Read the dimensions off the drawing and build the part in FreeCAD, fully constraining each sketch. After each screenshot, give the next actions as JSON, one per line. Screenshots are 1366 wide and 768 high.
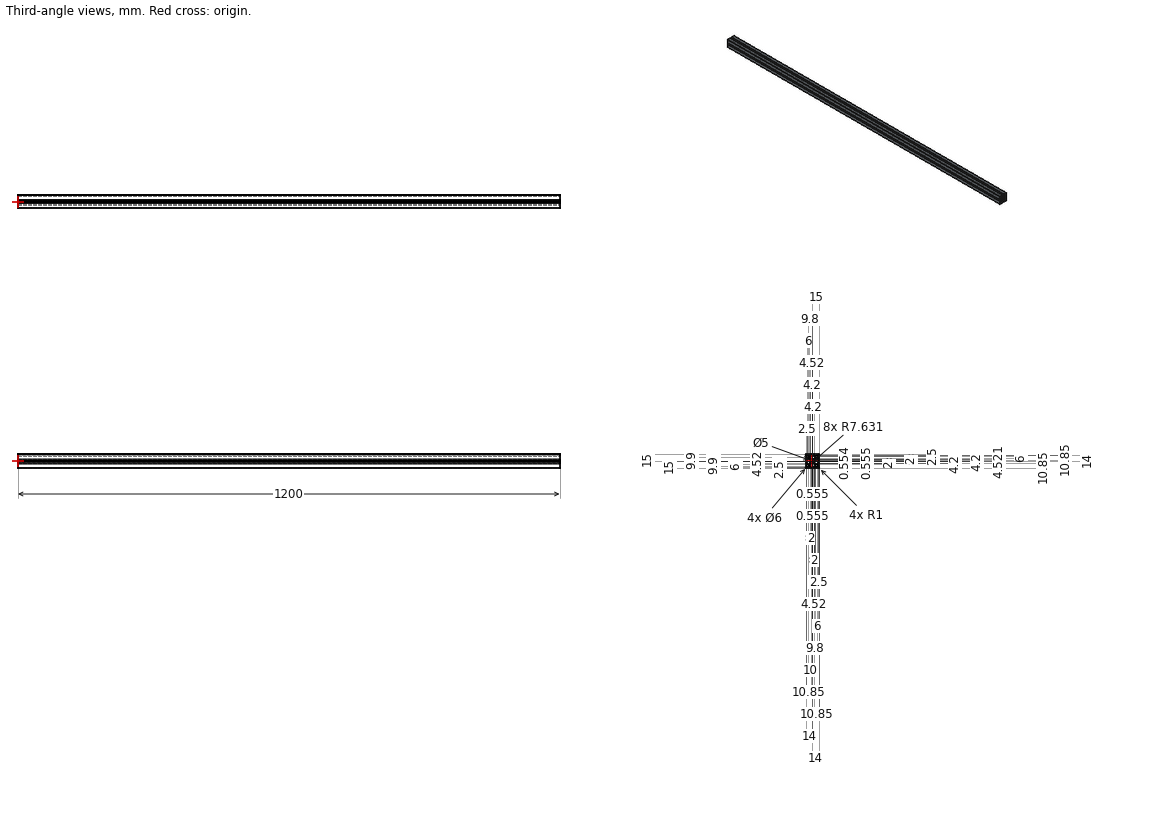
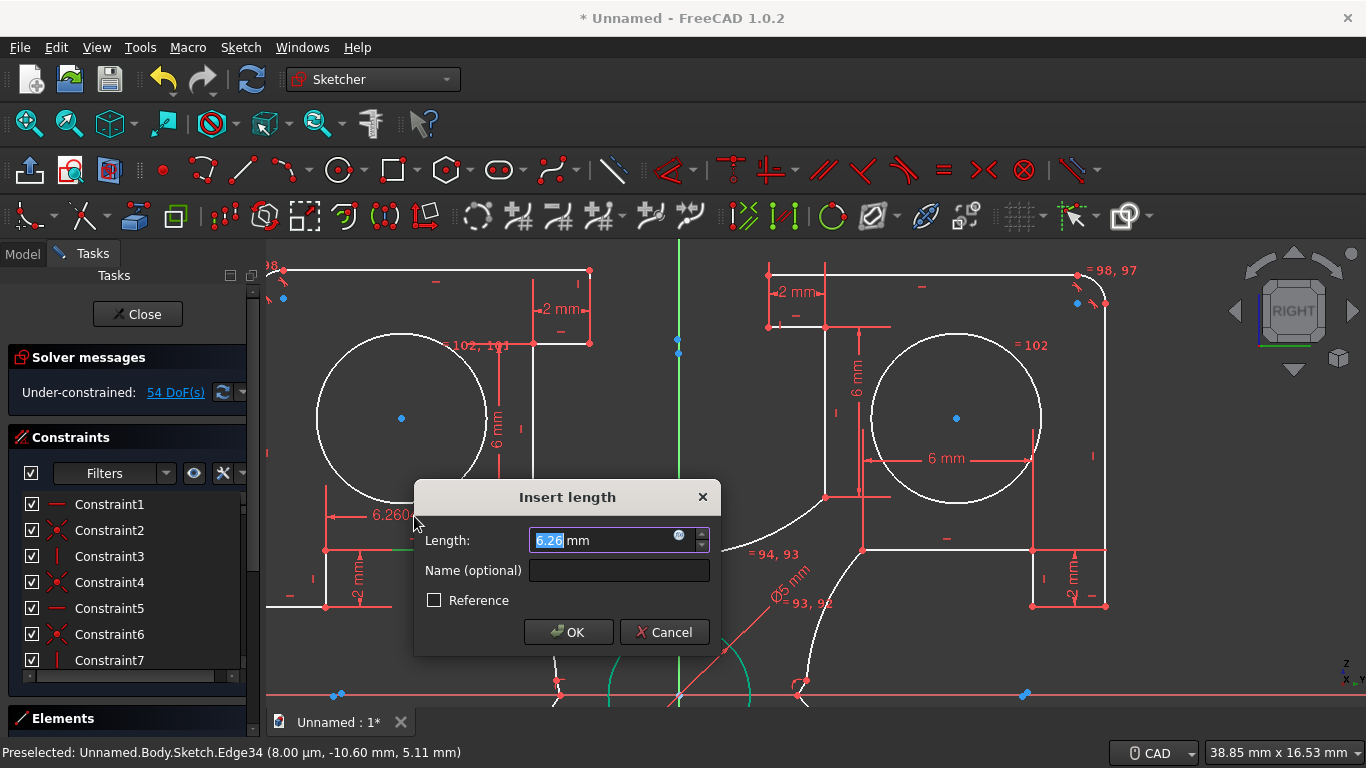
{"action": "type", "text": "6"}
{"action": "key", "text": "Return"}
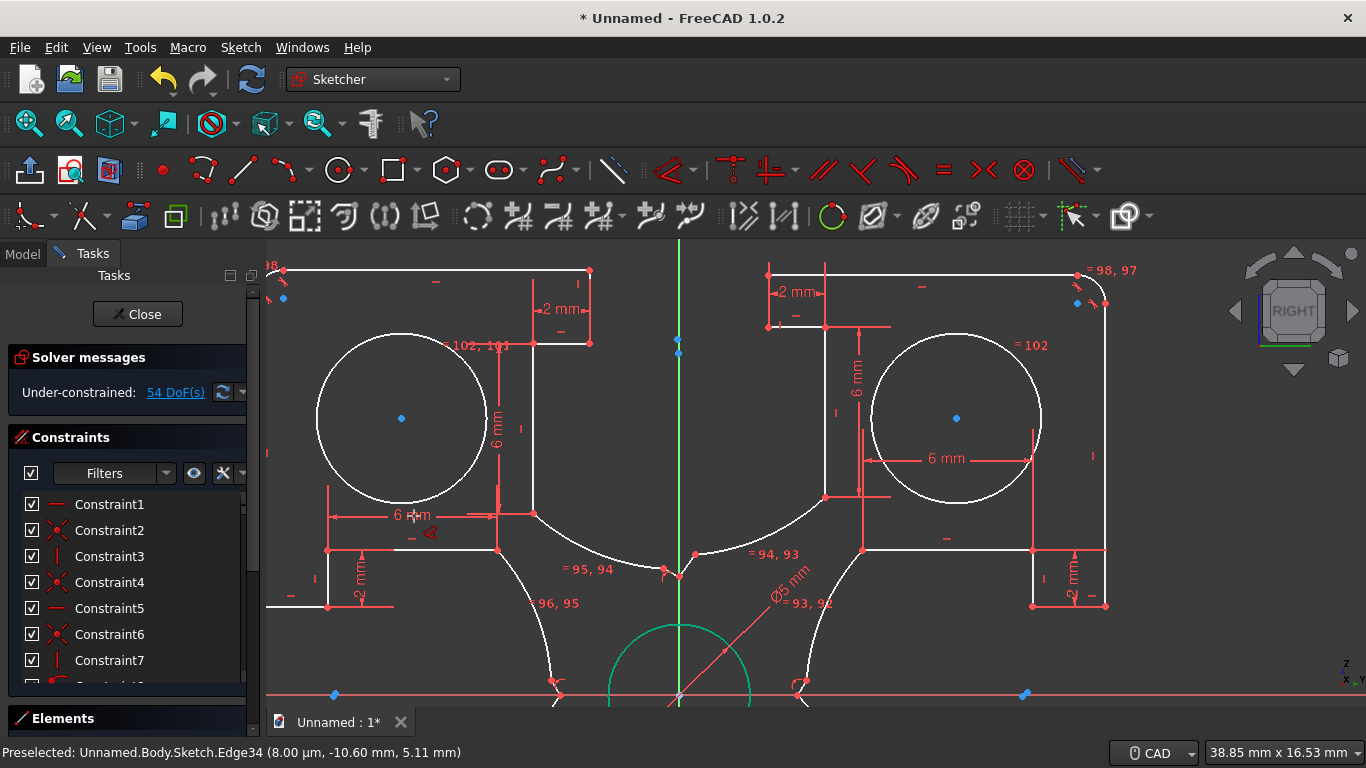
{"action": "scroll", "coordinate": [787, 344], "scroll_direction": "down", "scroll_amount": 5}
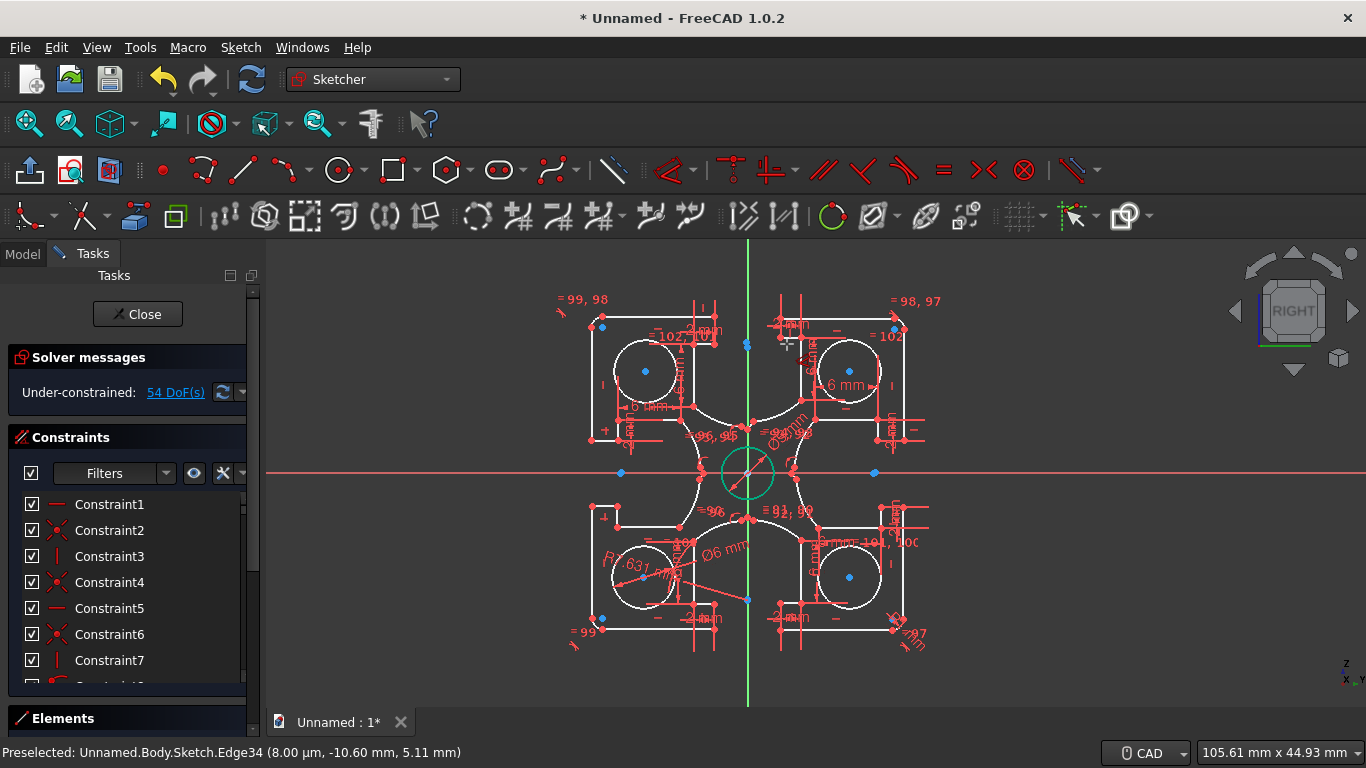
{"action": "left_click", "coordinate": [661, 527]}
{"action": "left_click", "coordinate": [648, 493]}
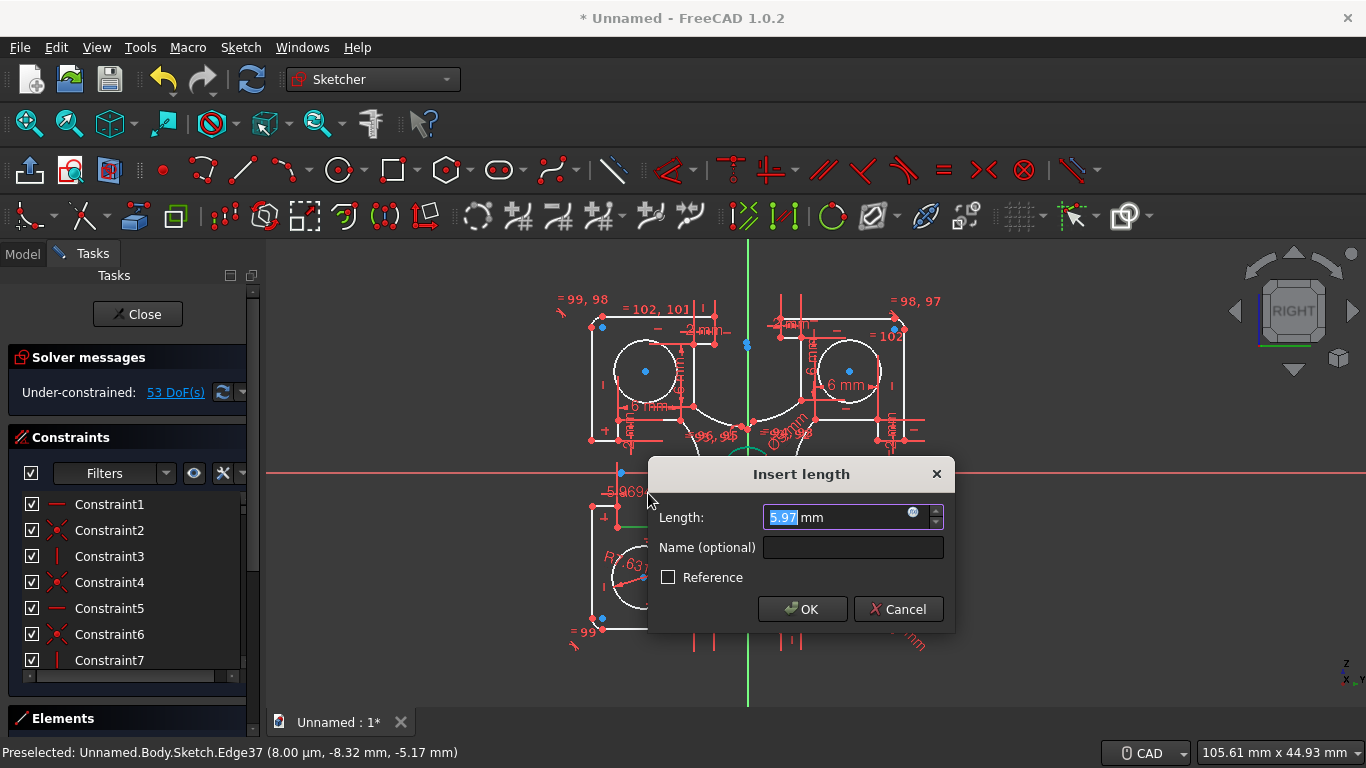
{"action": "type", "text": "6"}
{"action": "key", "text": "Return"}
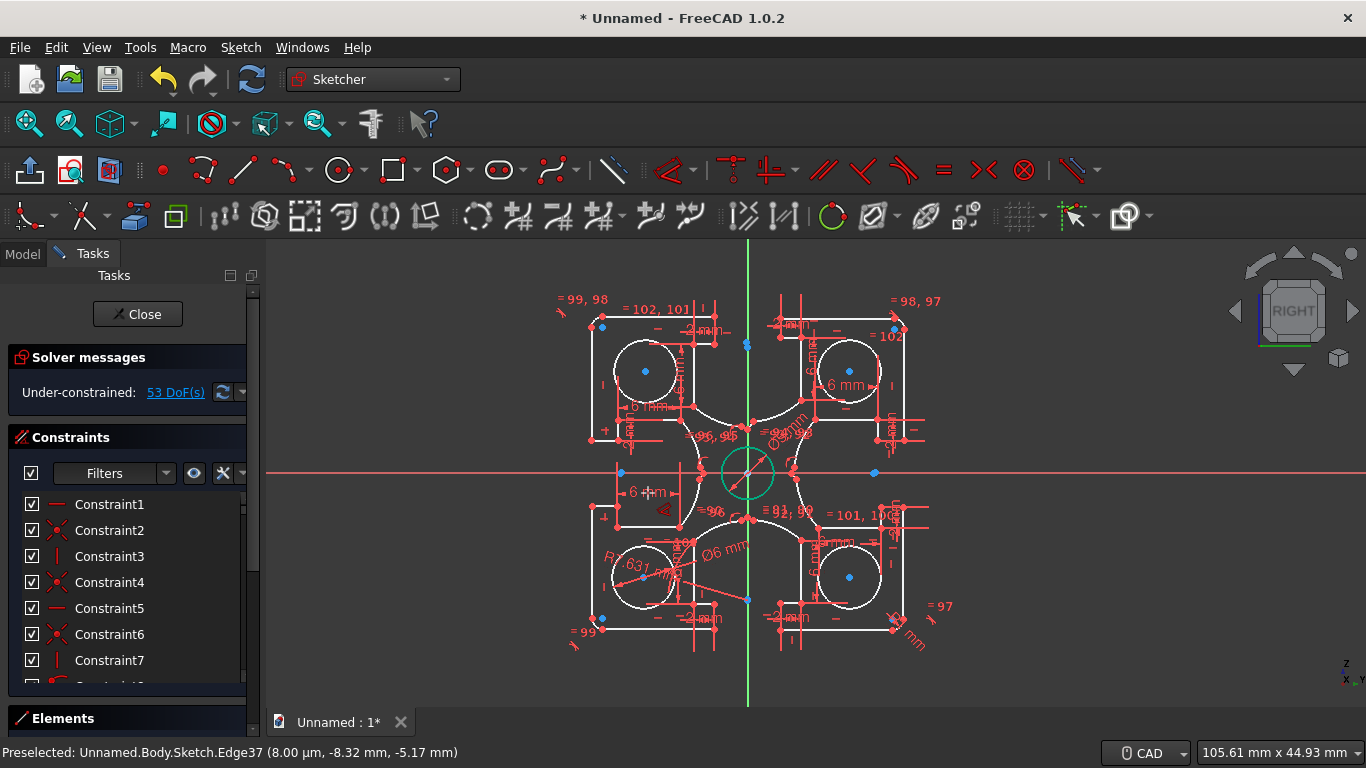
{"action": "scroll", "coordinate": [617, 517], "scroll_direction": "up", "scroll_amount": 4}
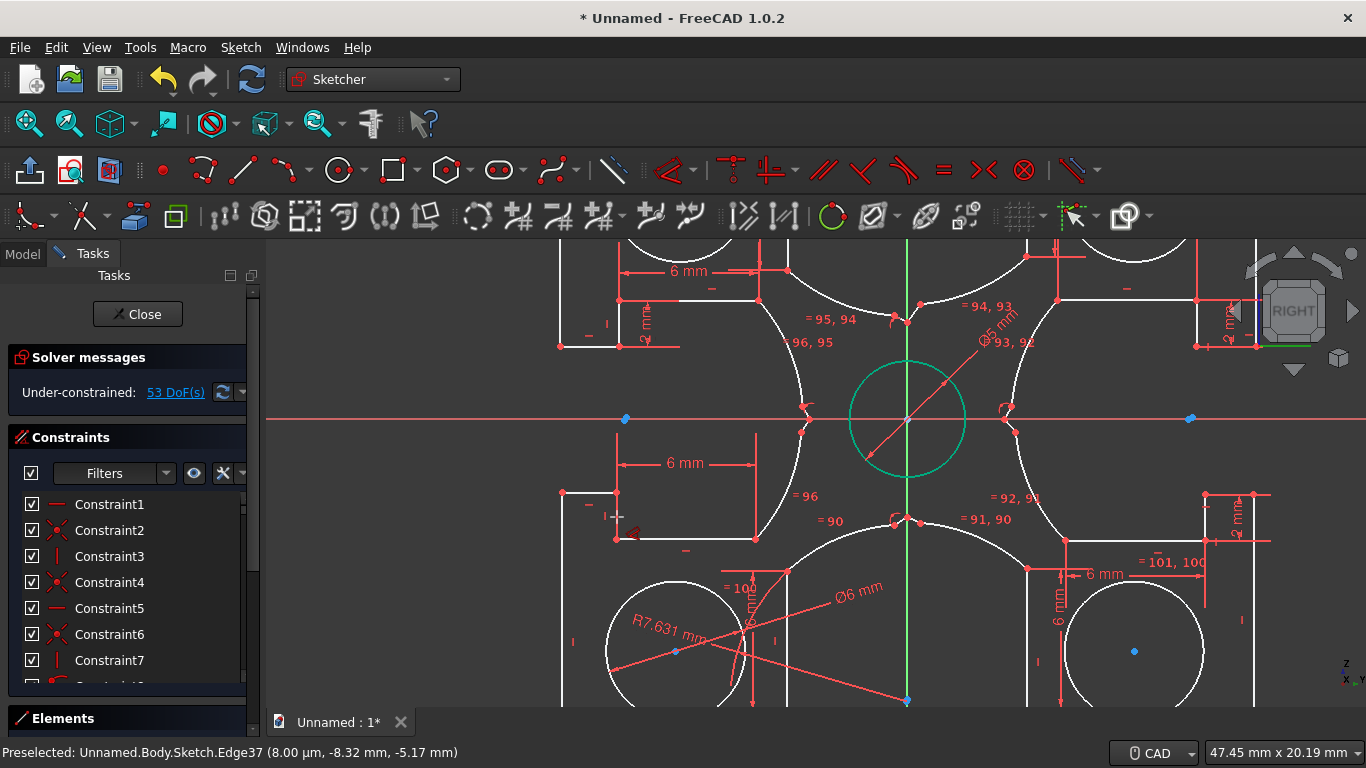
{"action": "left_click", "coordinate": [617, 516]}
{"action": "left_click", "coordinate": [583, 516]}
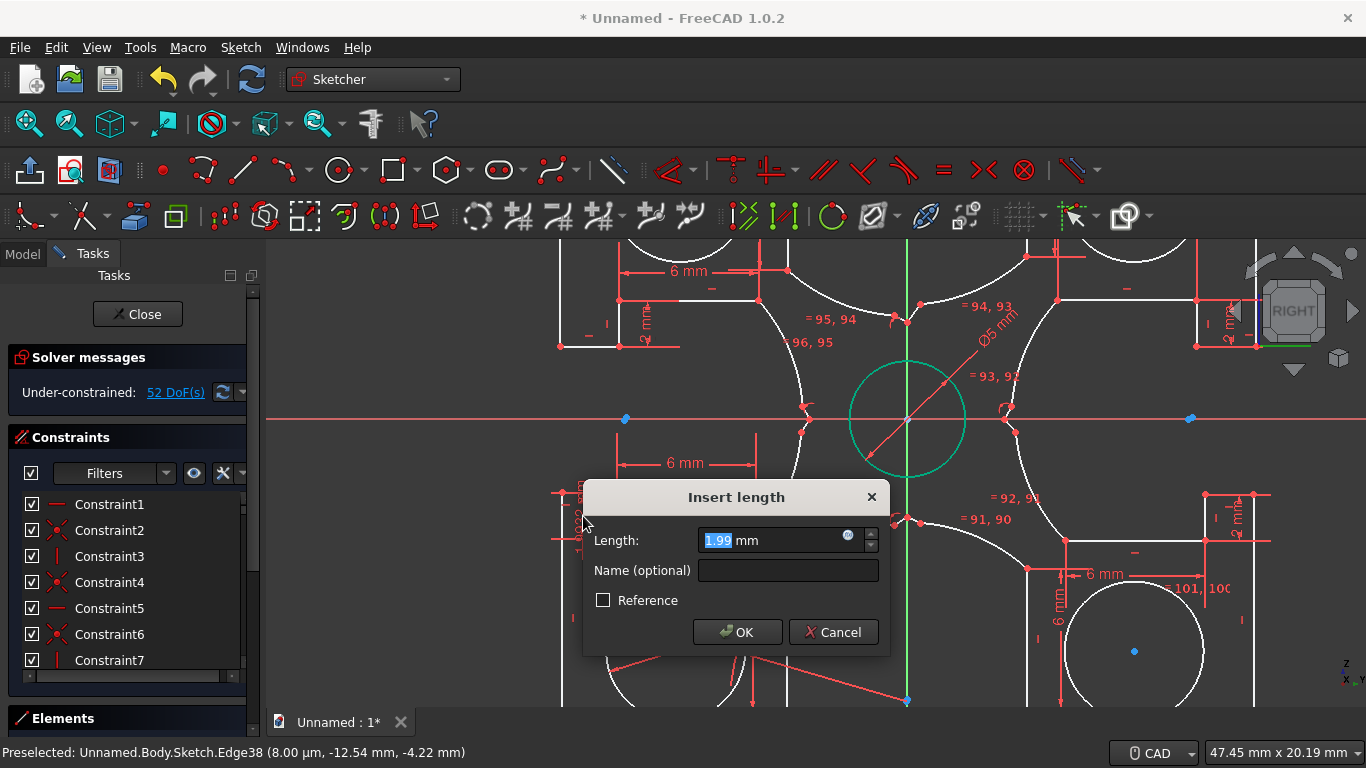
{"action": "type", "text": "2"}
{"action": "key", "text": "Return"}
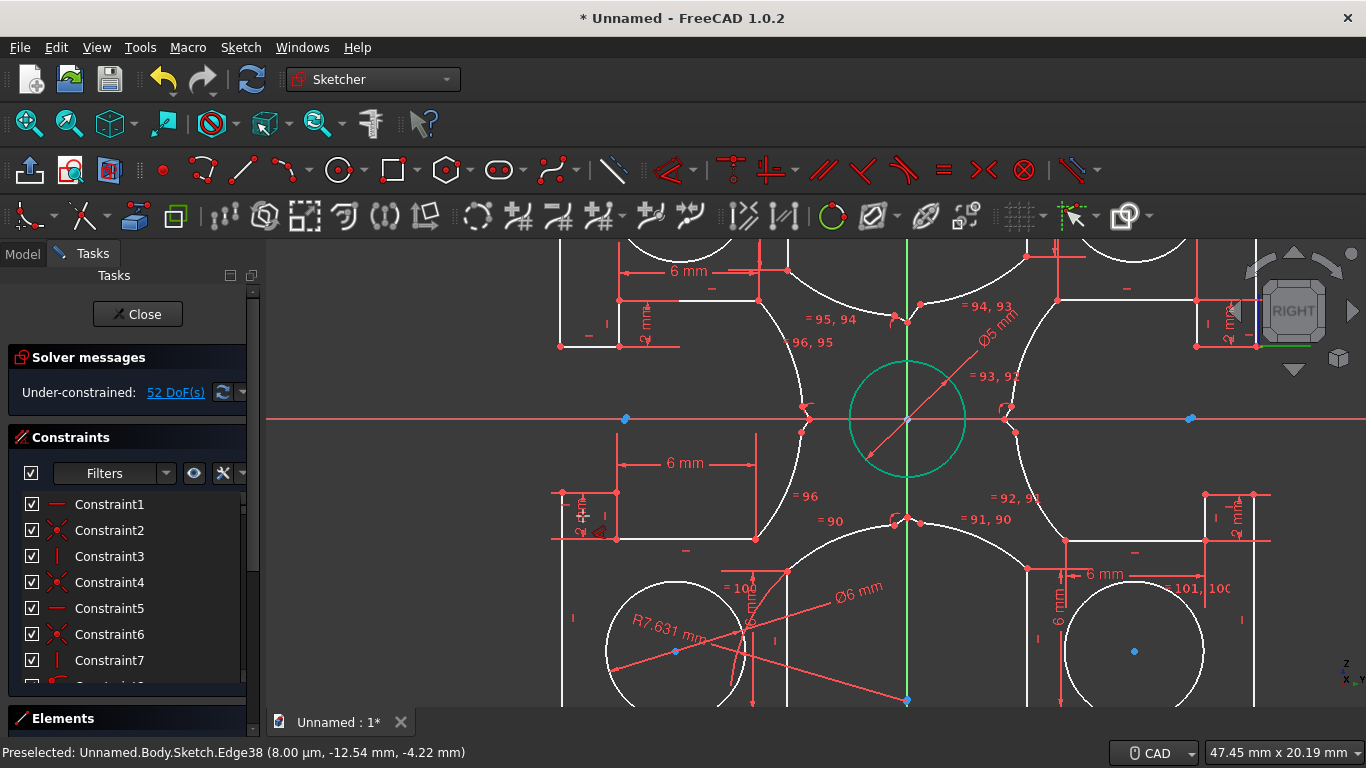
{"action": "left_click", "coordinate": [676, 651]}
{"action": "left_click", "coordinate": [738, 385]}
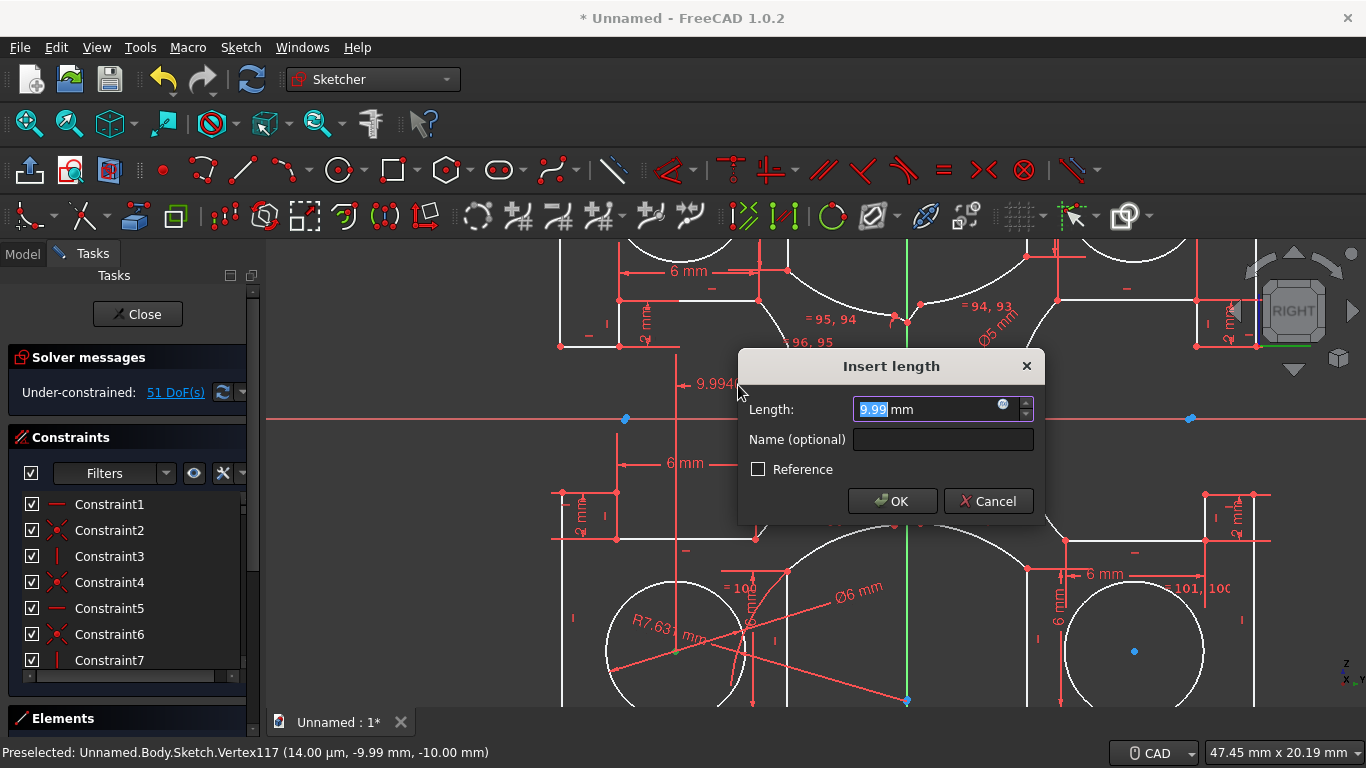
{"action": "type", "text": "10"}
{"action": "key", "text": "Return"}